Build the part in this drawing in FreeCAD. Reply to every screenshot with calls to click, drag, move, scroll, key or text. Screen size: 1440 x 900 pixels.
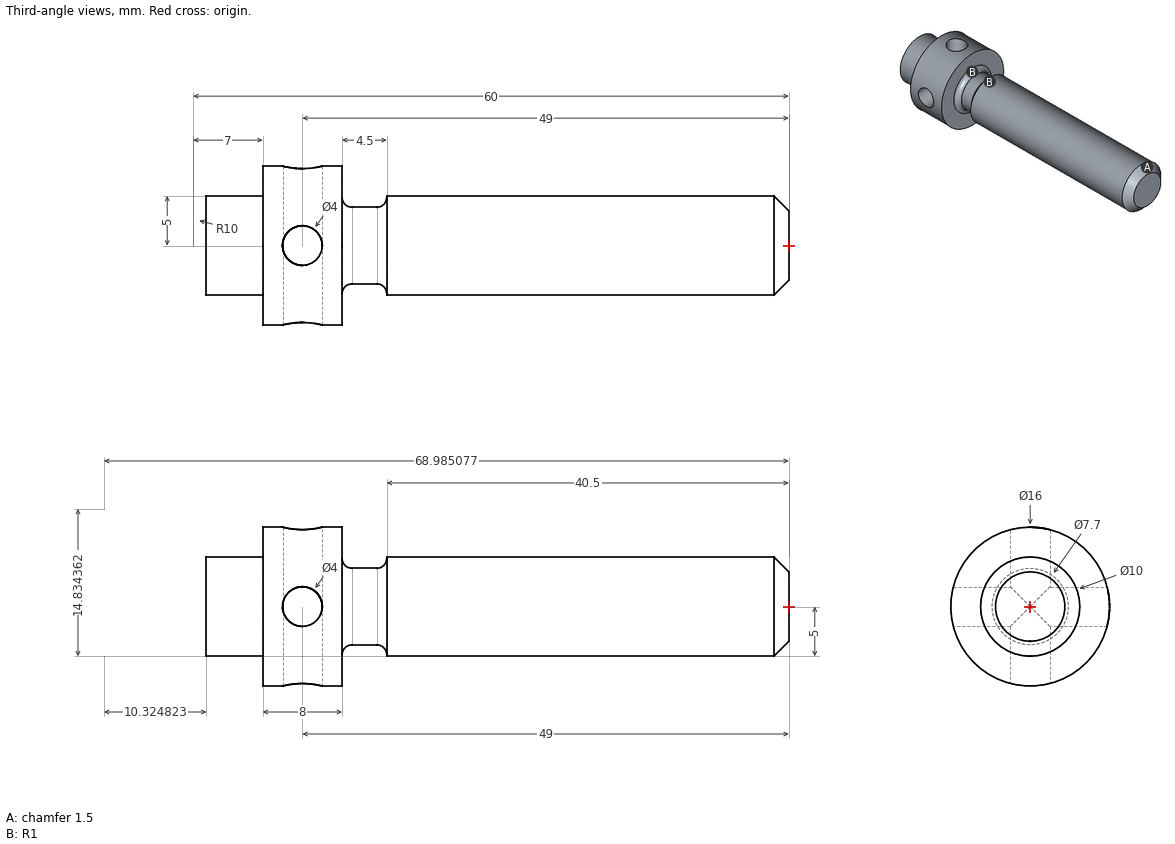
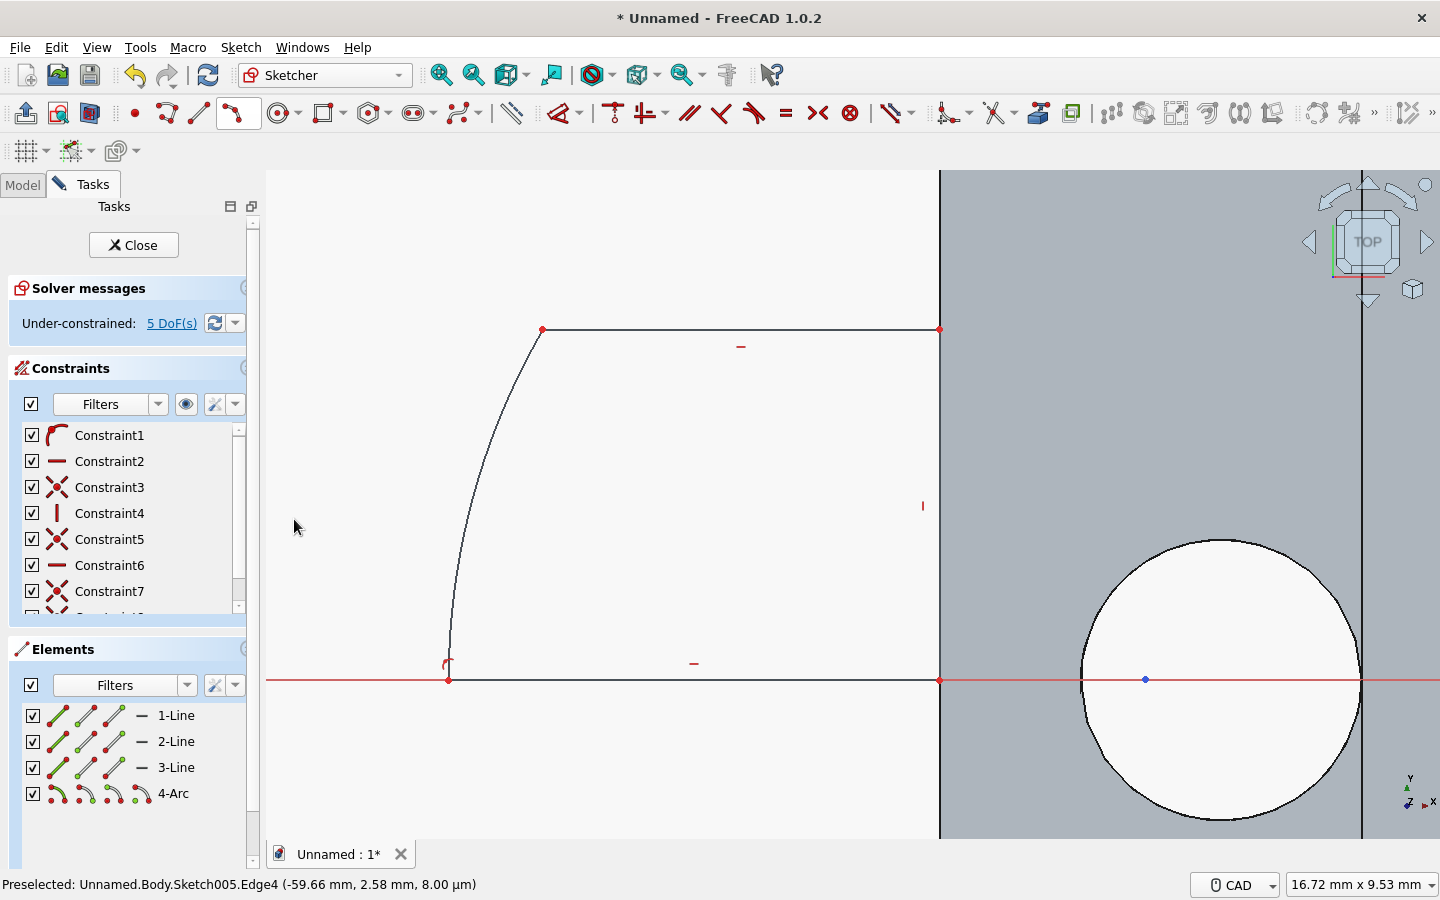
click(1146, 680)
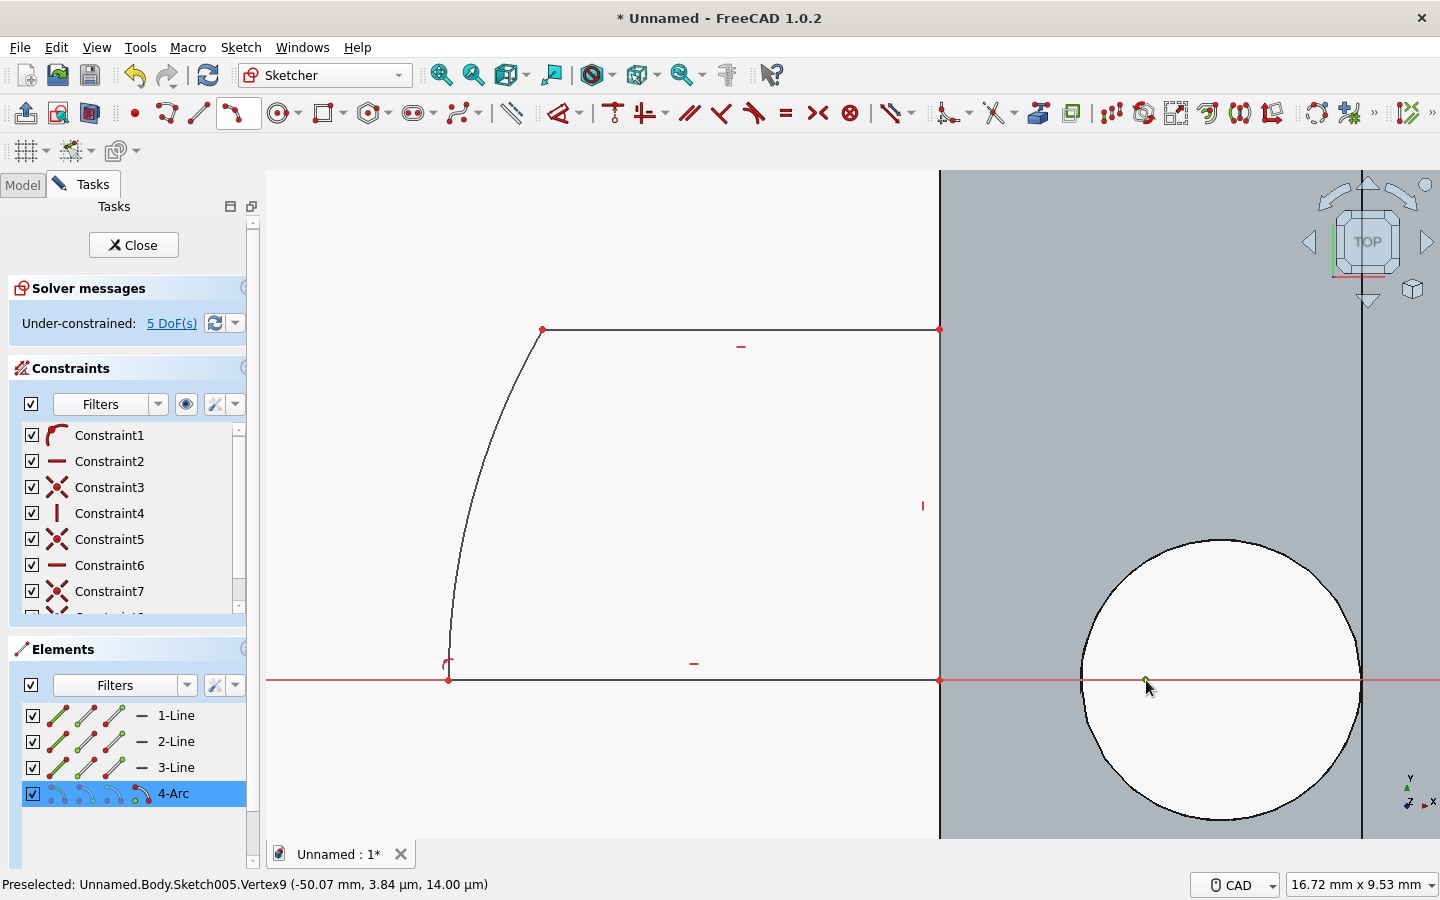
click(364, 680)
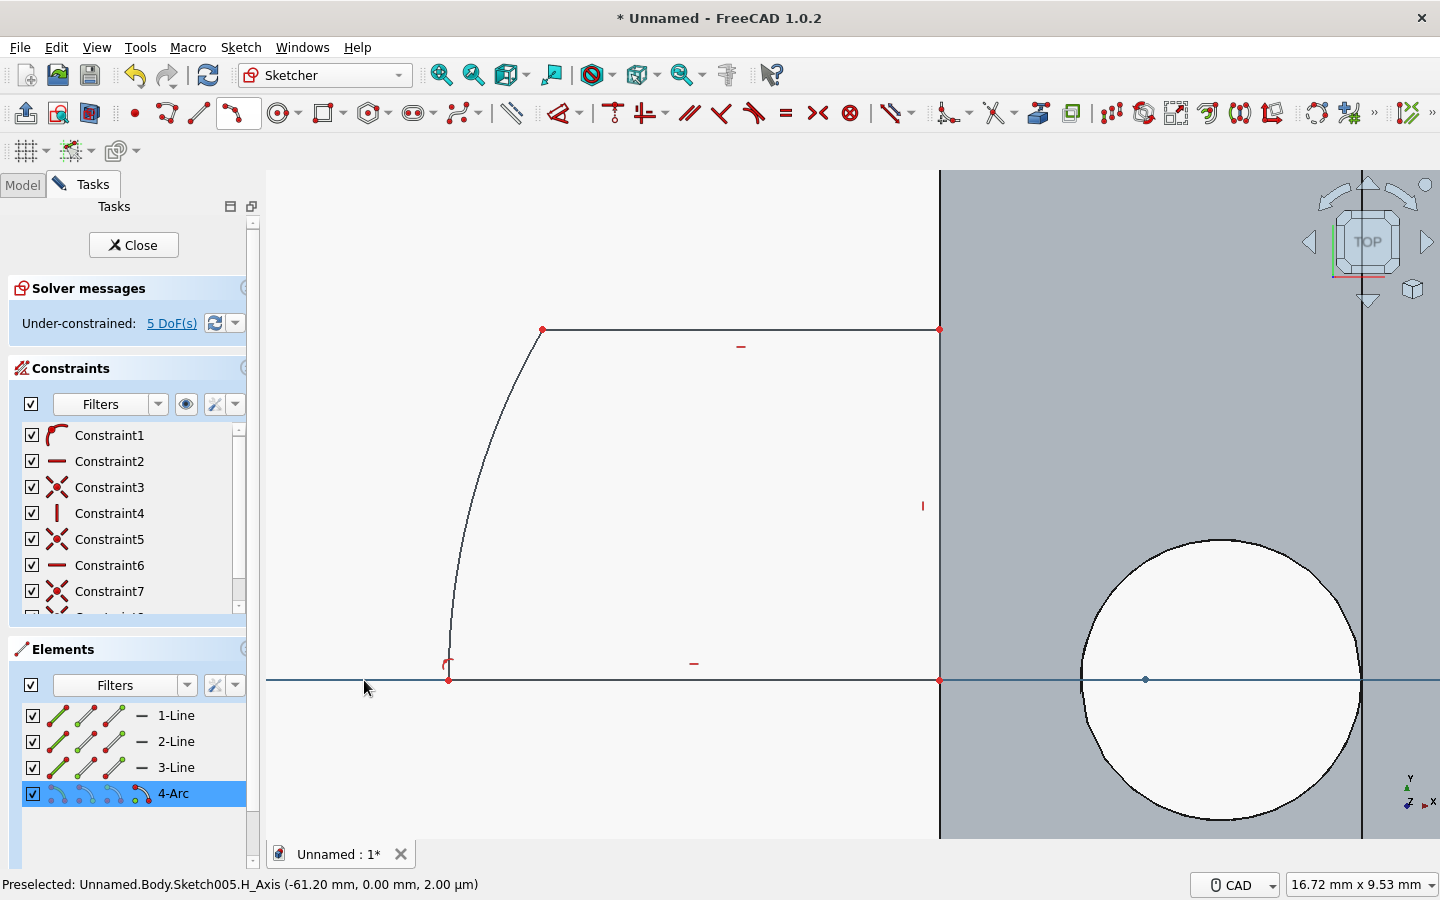
click(614, 114)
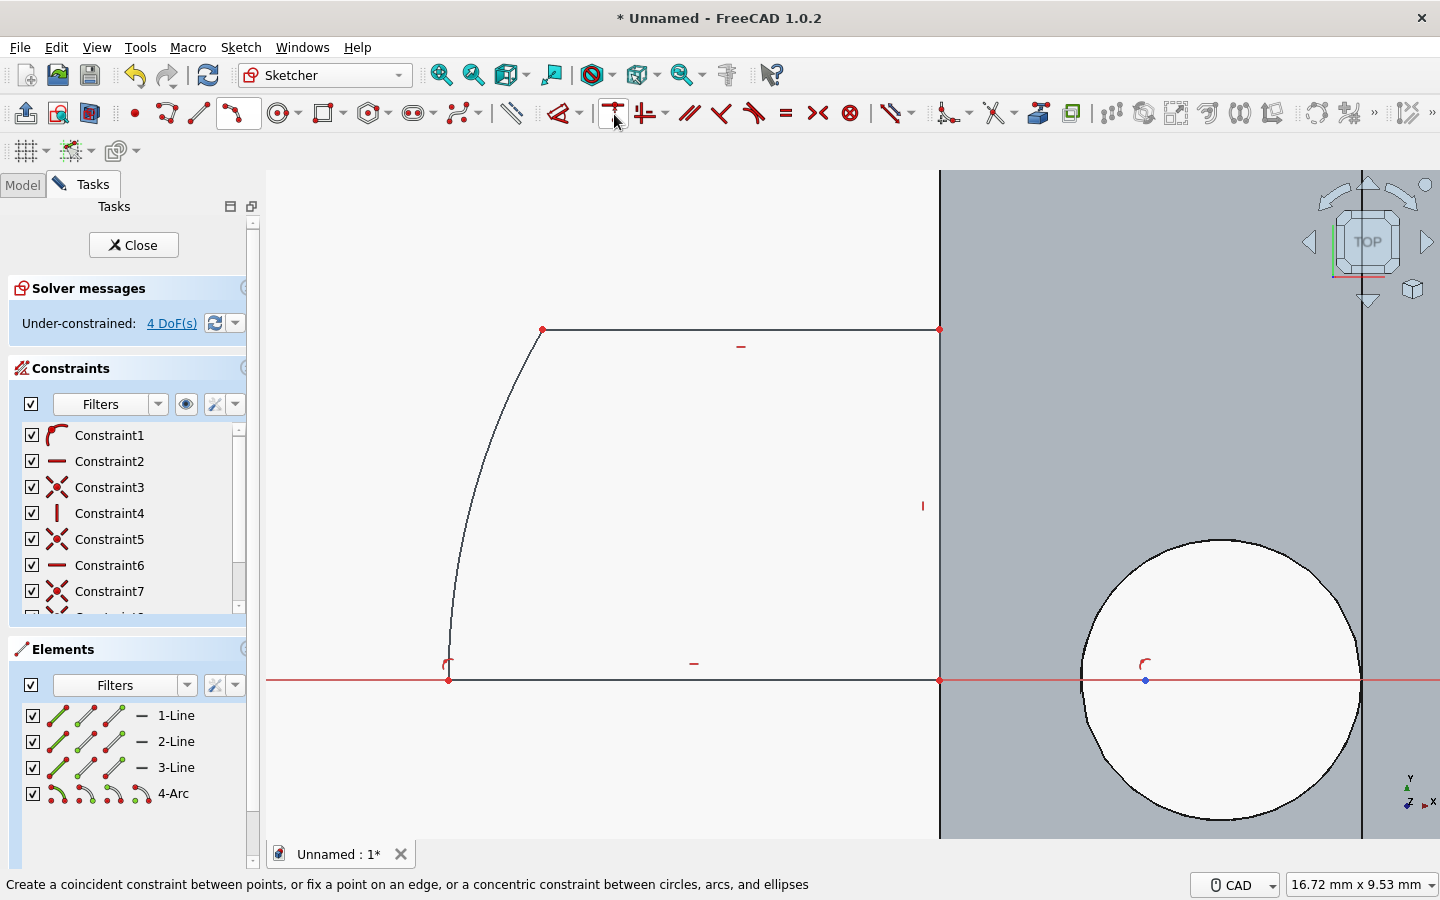
click(558, 114)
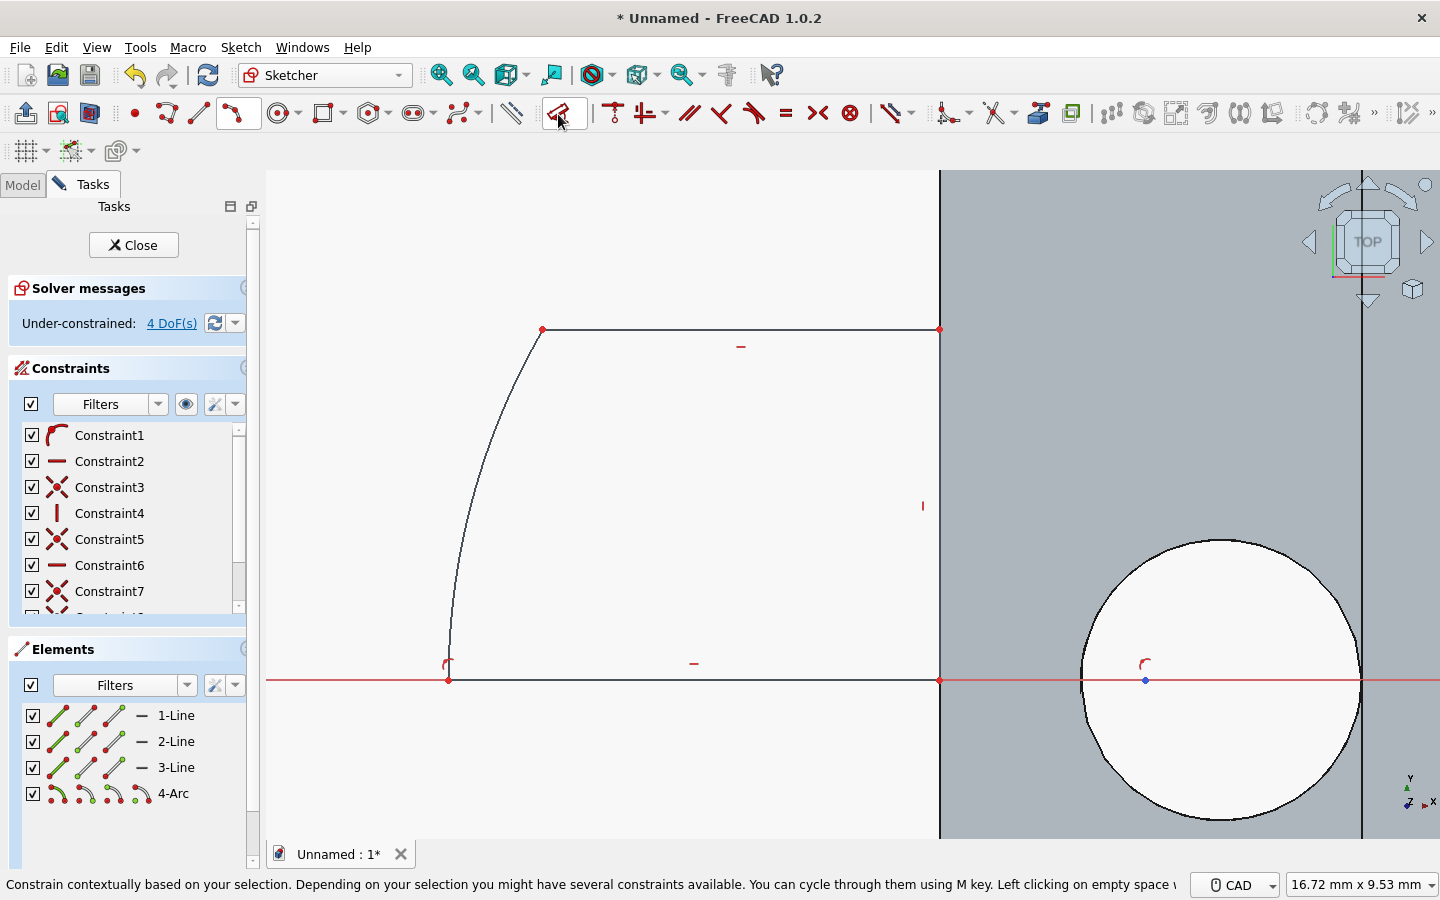
click(495, 429)
click(465, 417)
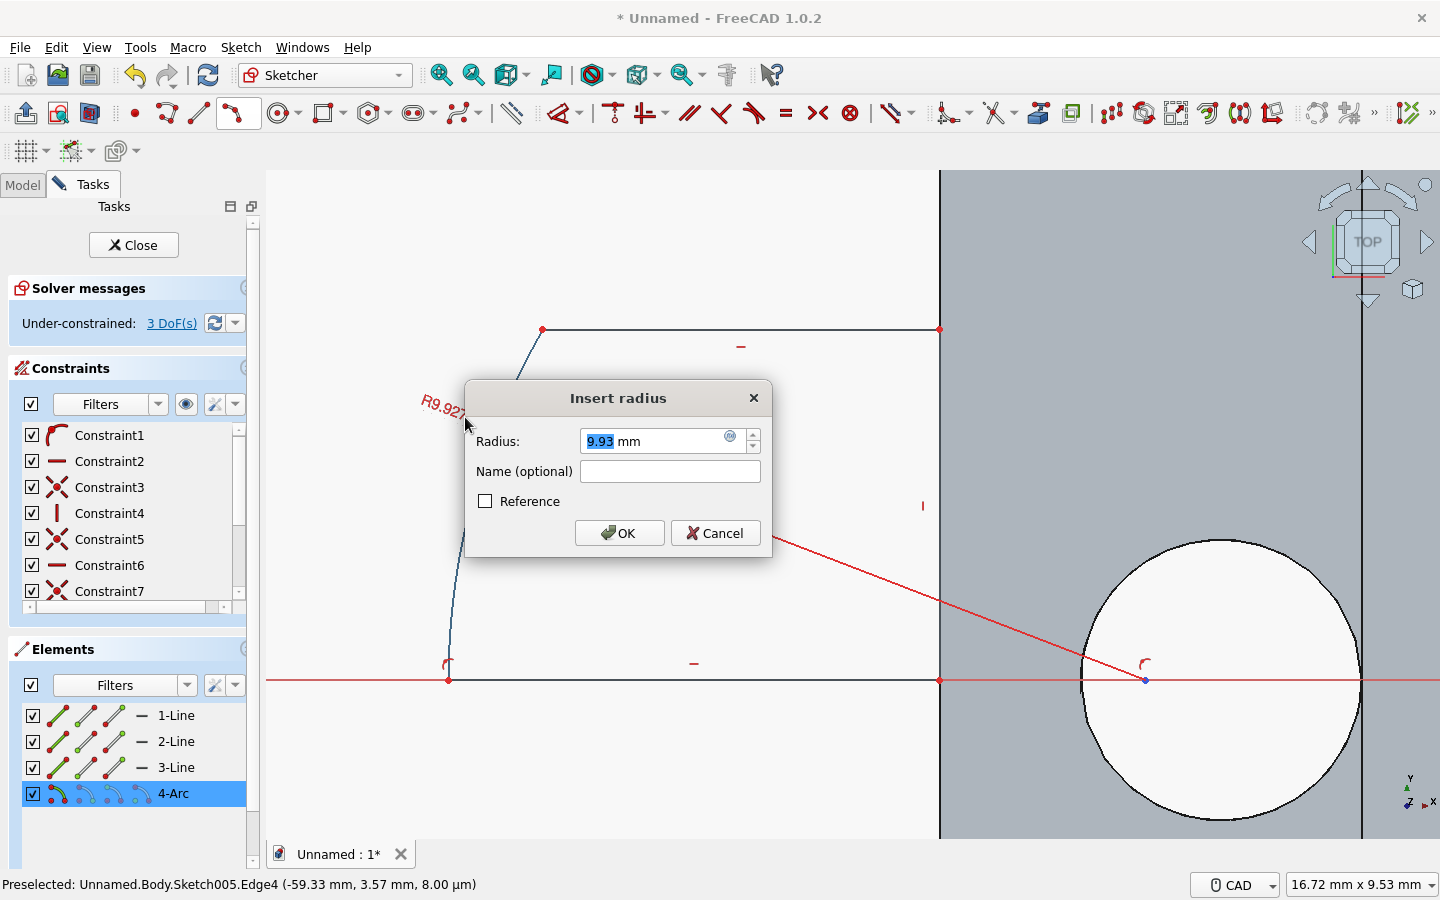
text(10)
key(Return)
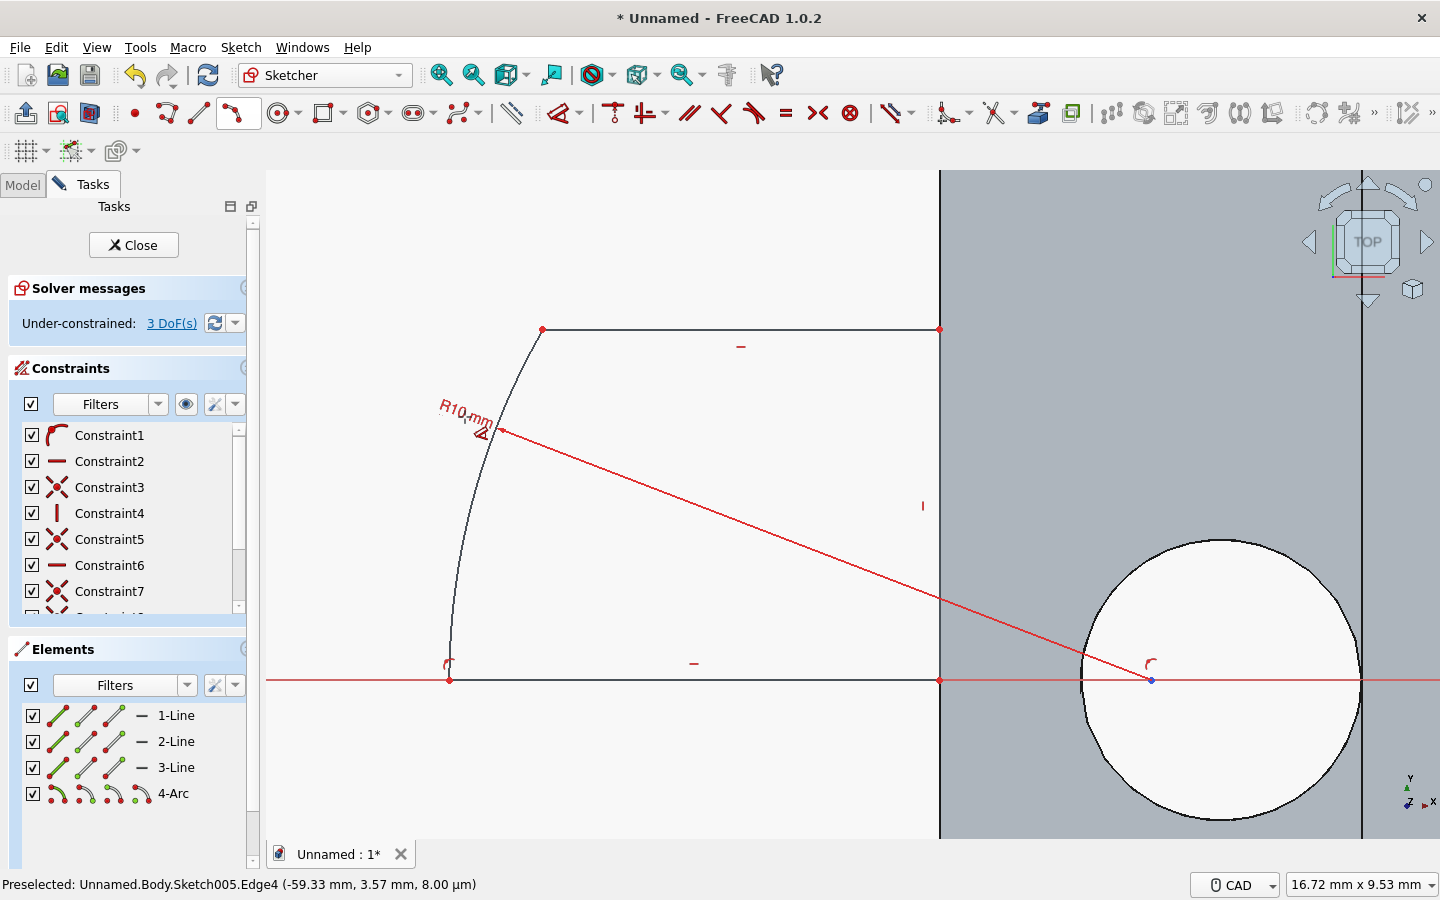
click(597, 680)
click(695, 714)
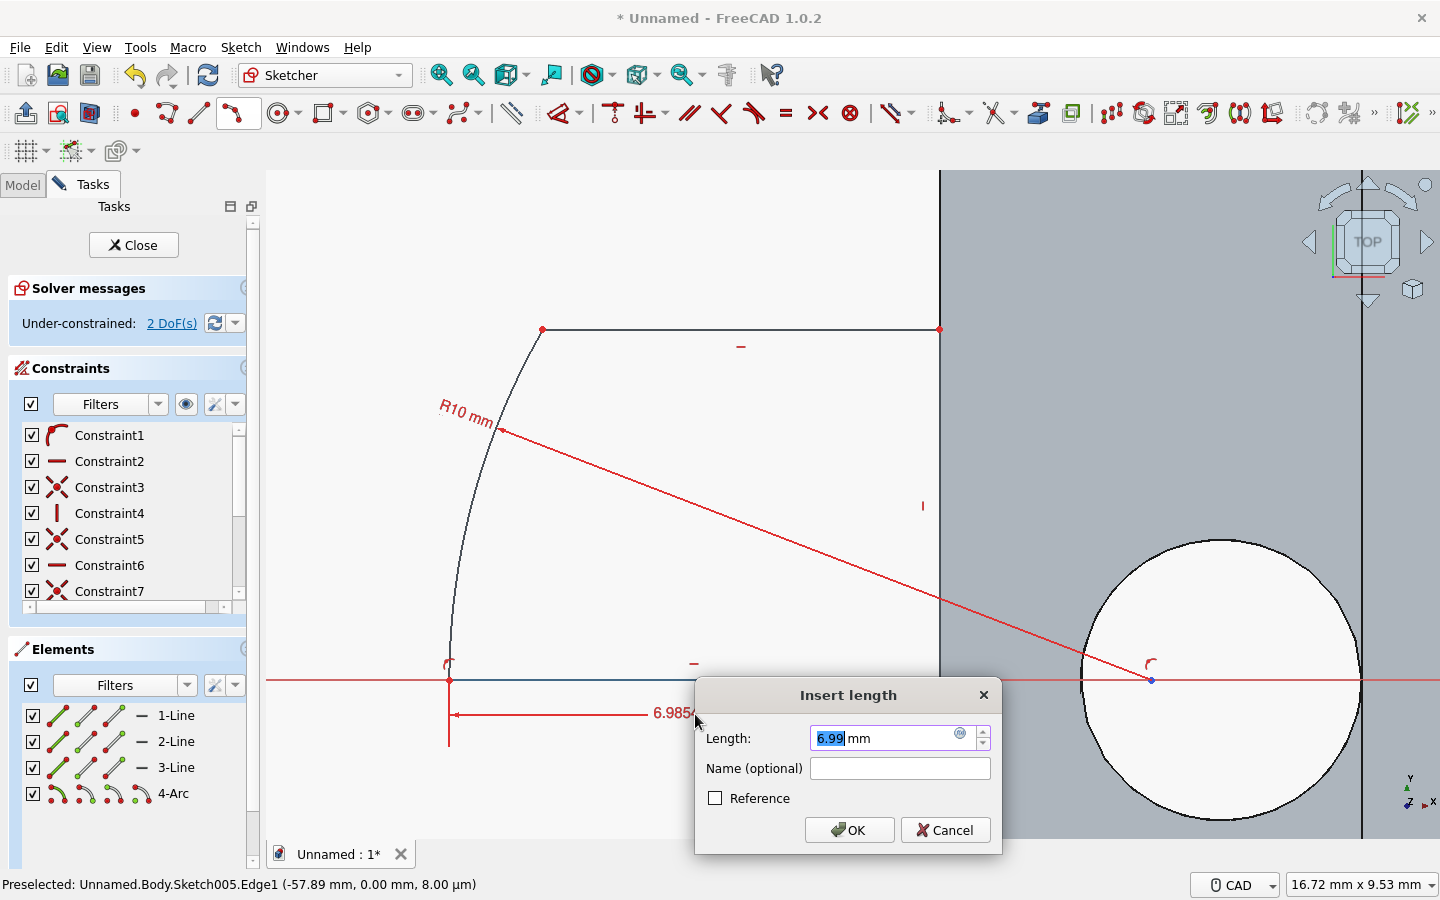
text(7)
key(Return)